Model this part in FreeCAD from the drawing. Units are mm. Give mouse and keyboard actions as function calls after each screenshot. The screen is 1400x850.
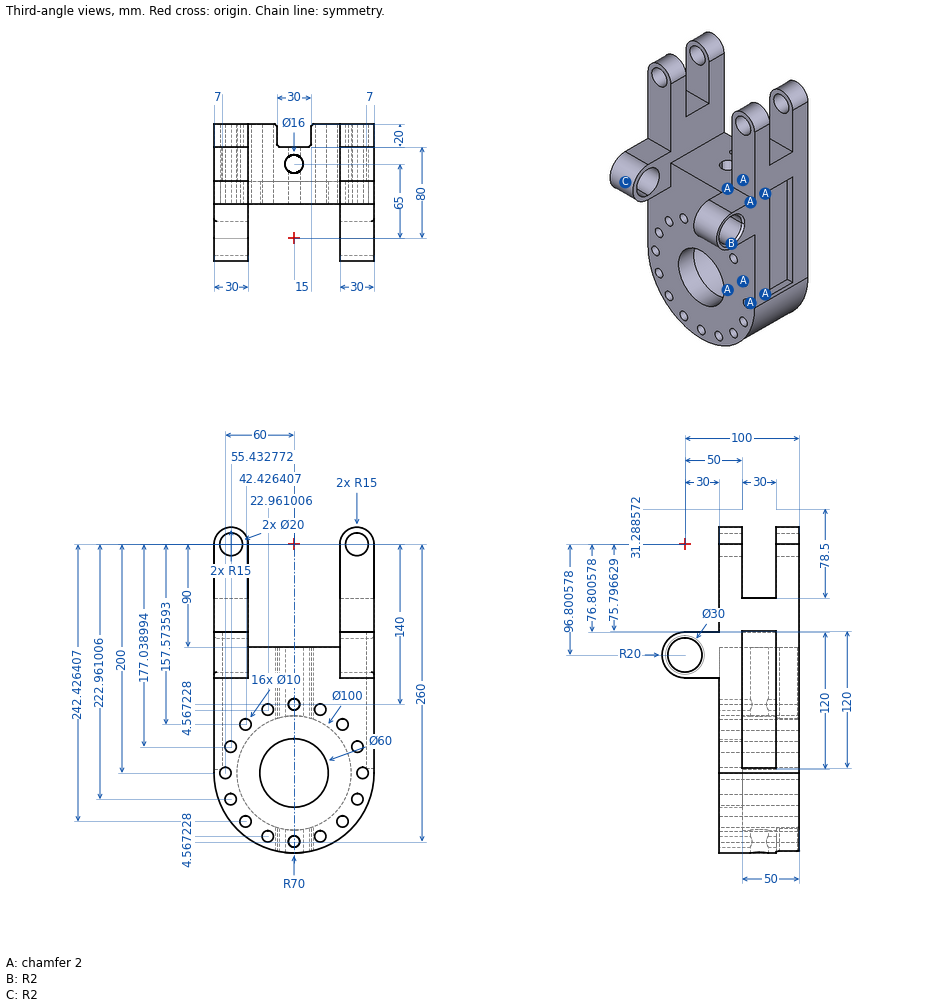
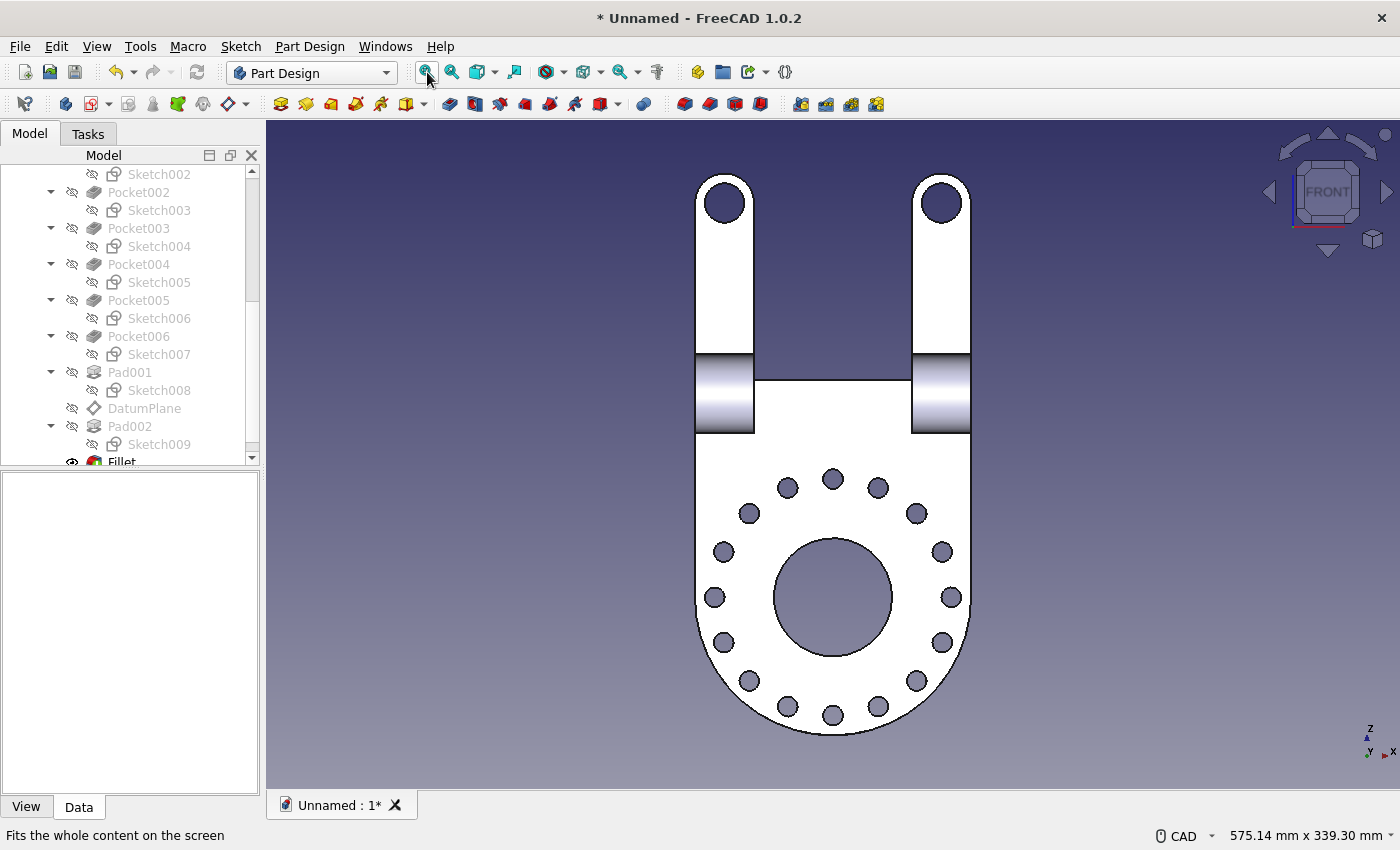
key(3)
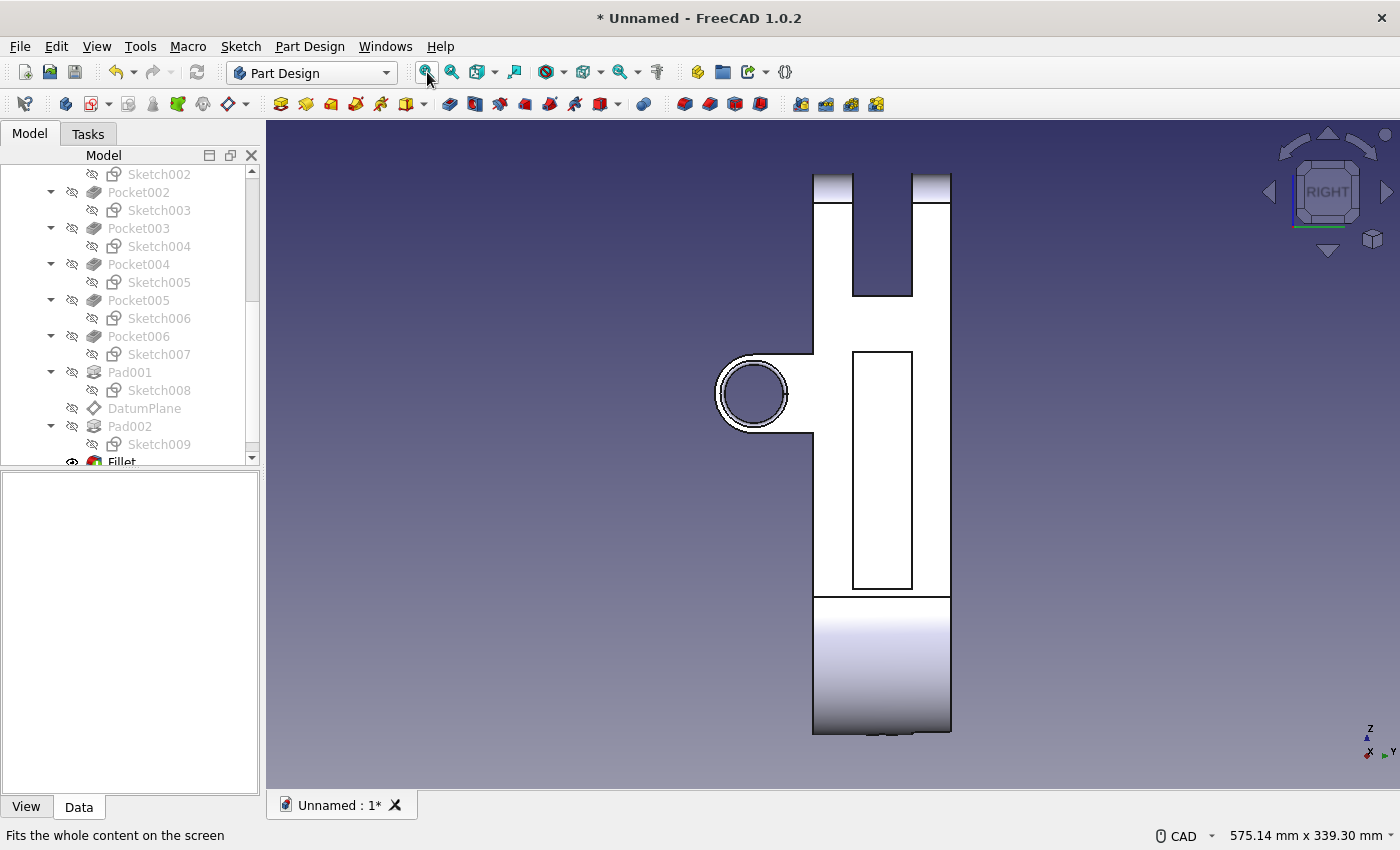
key(5)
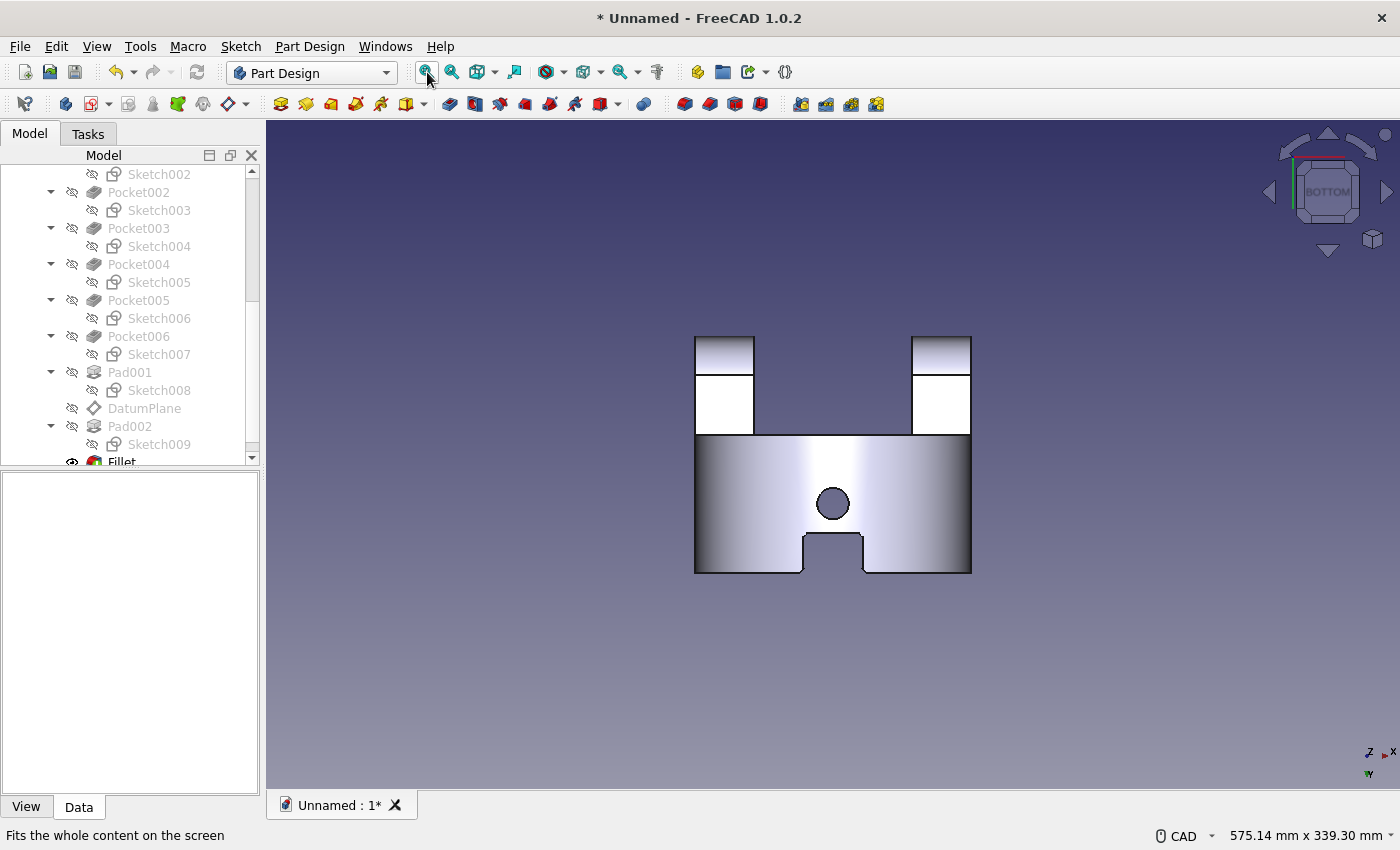
key(v)
key(f)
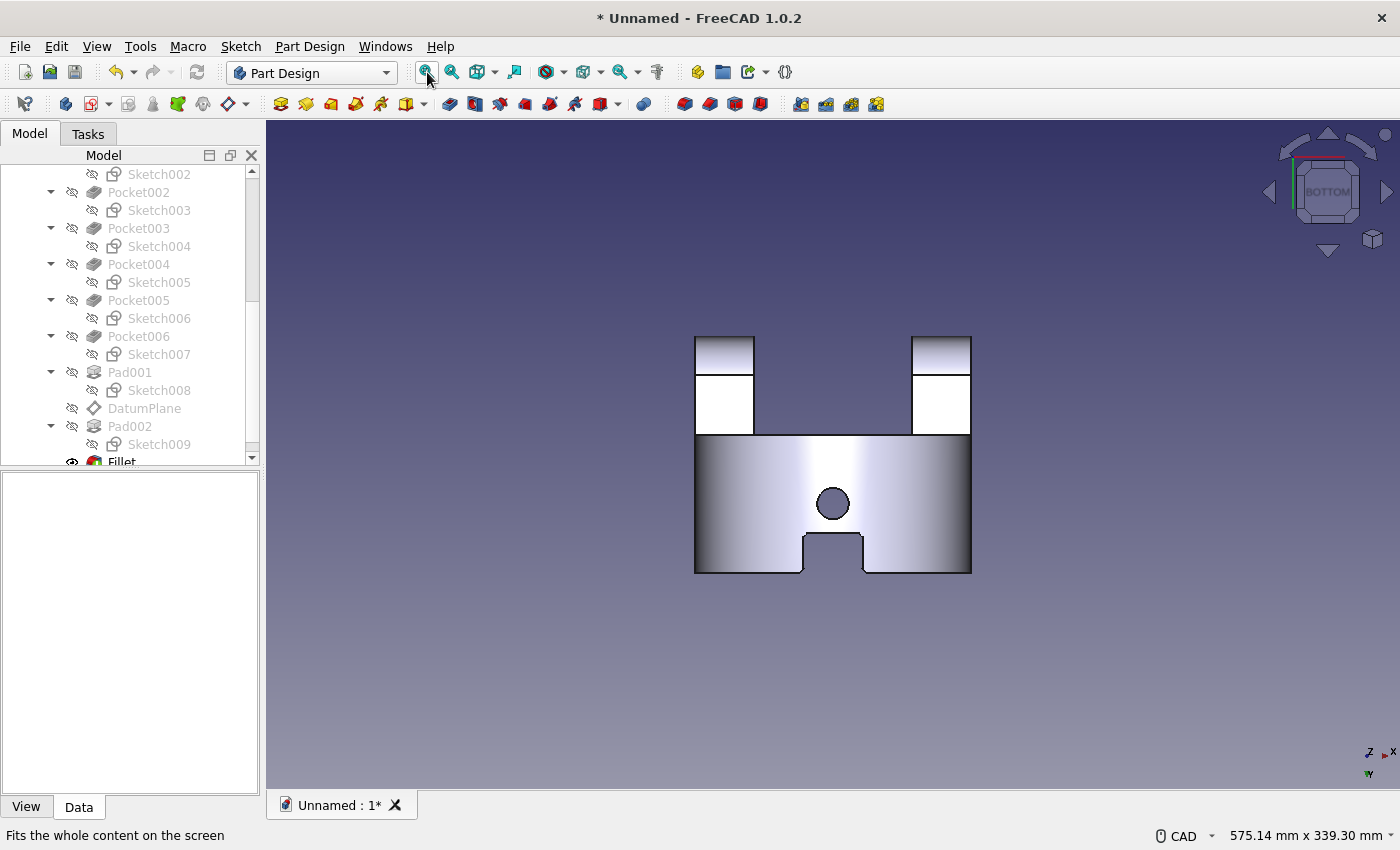
key(4)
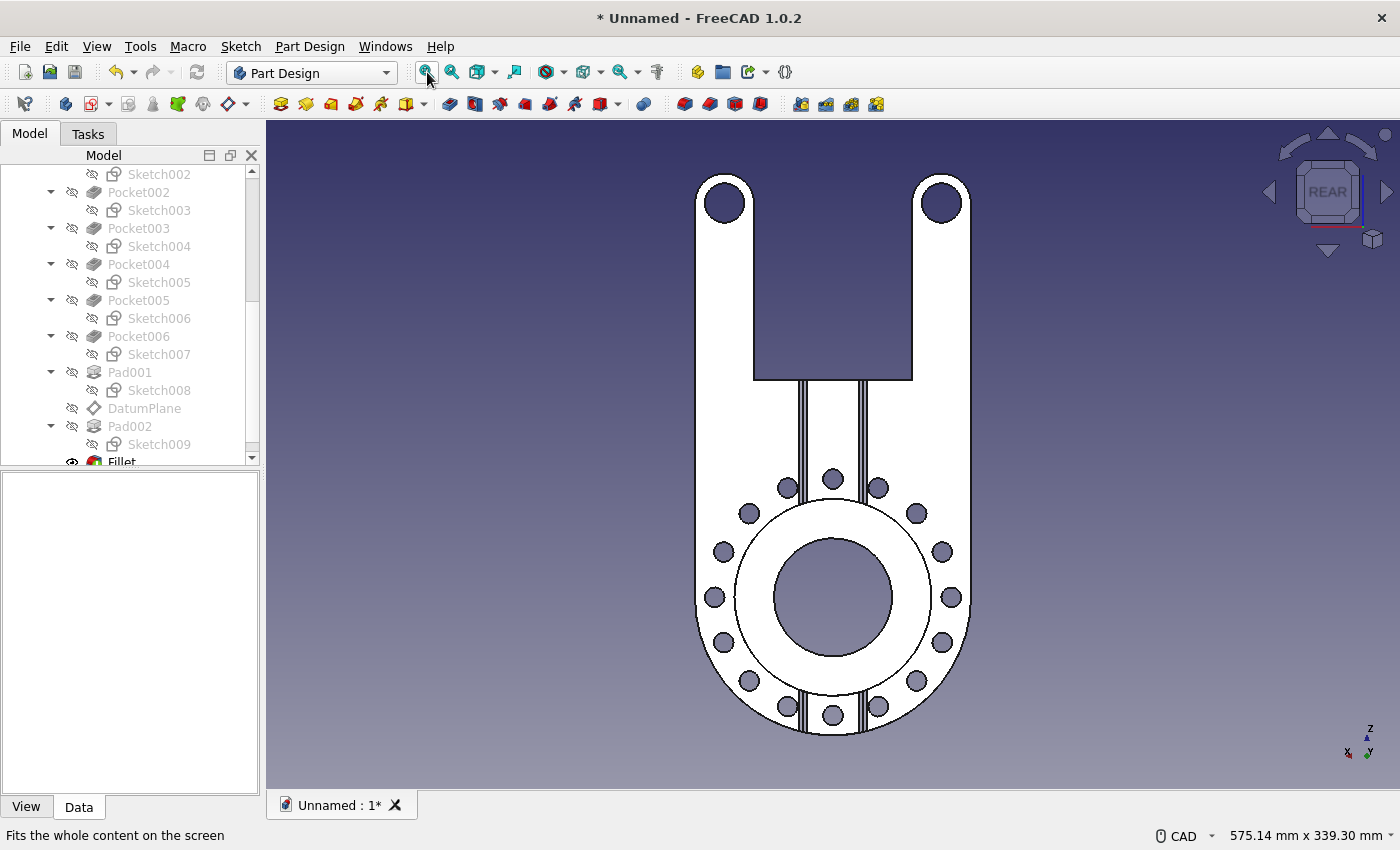
key(6)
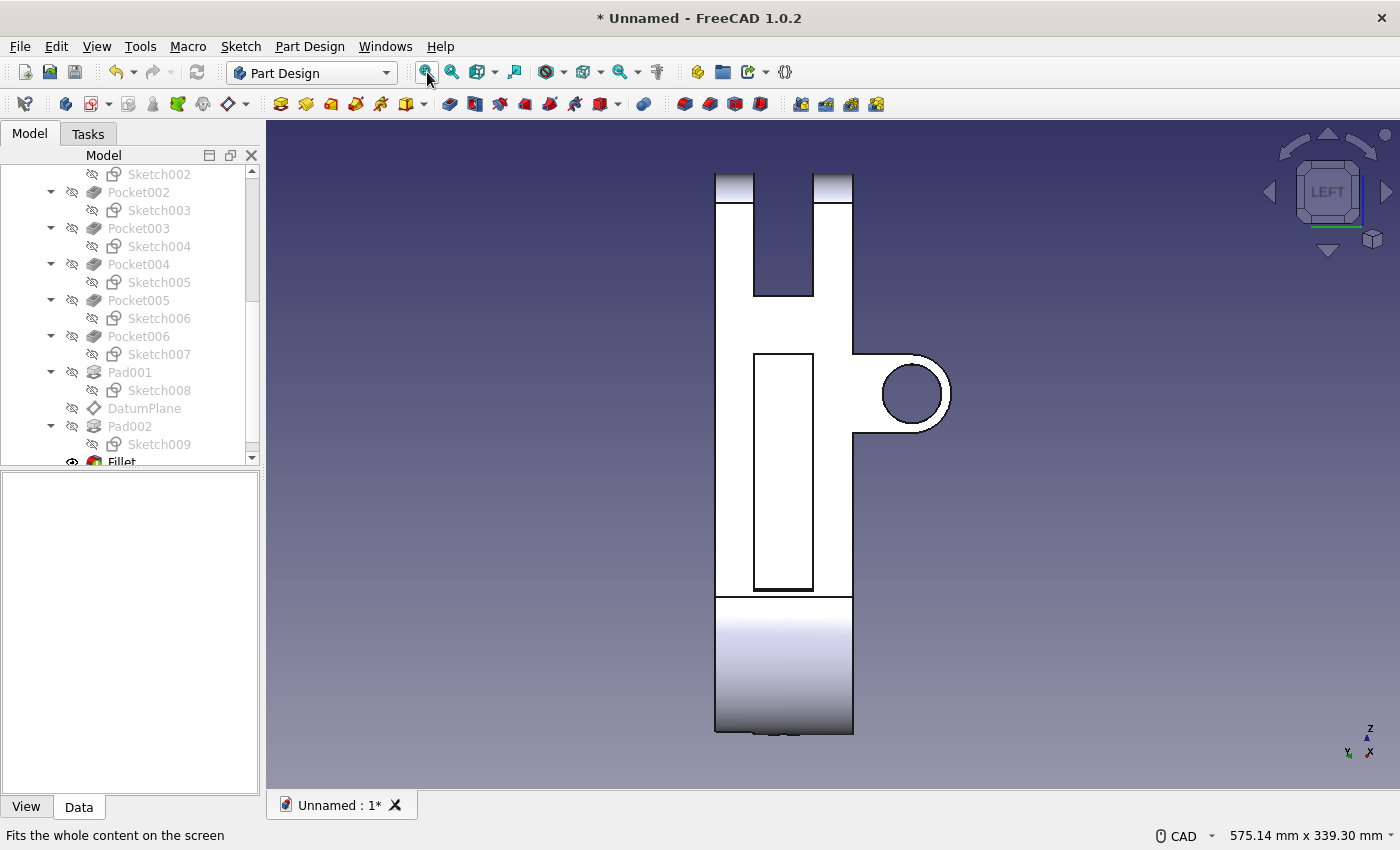
click(912, 363)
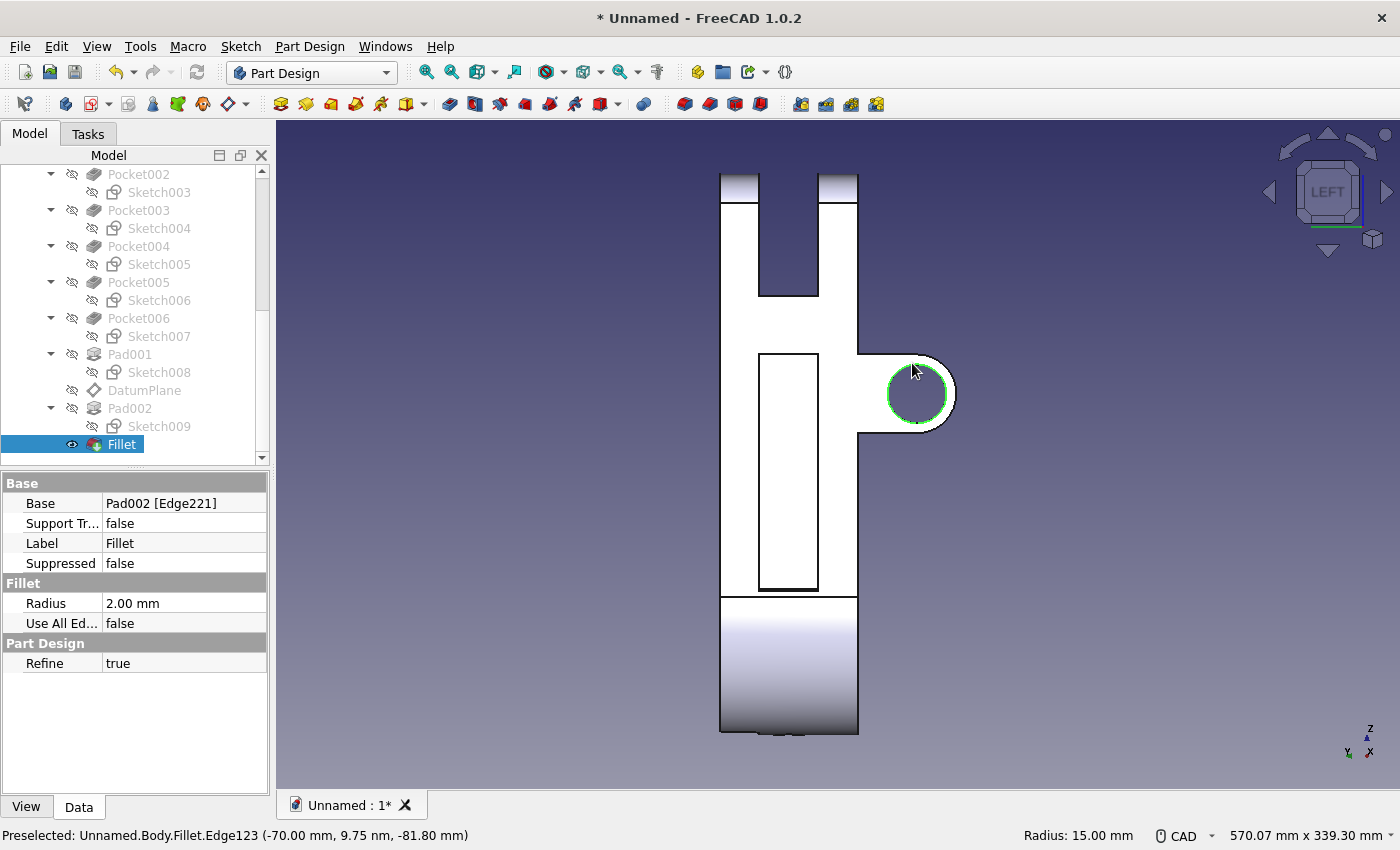
click(685, 104)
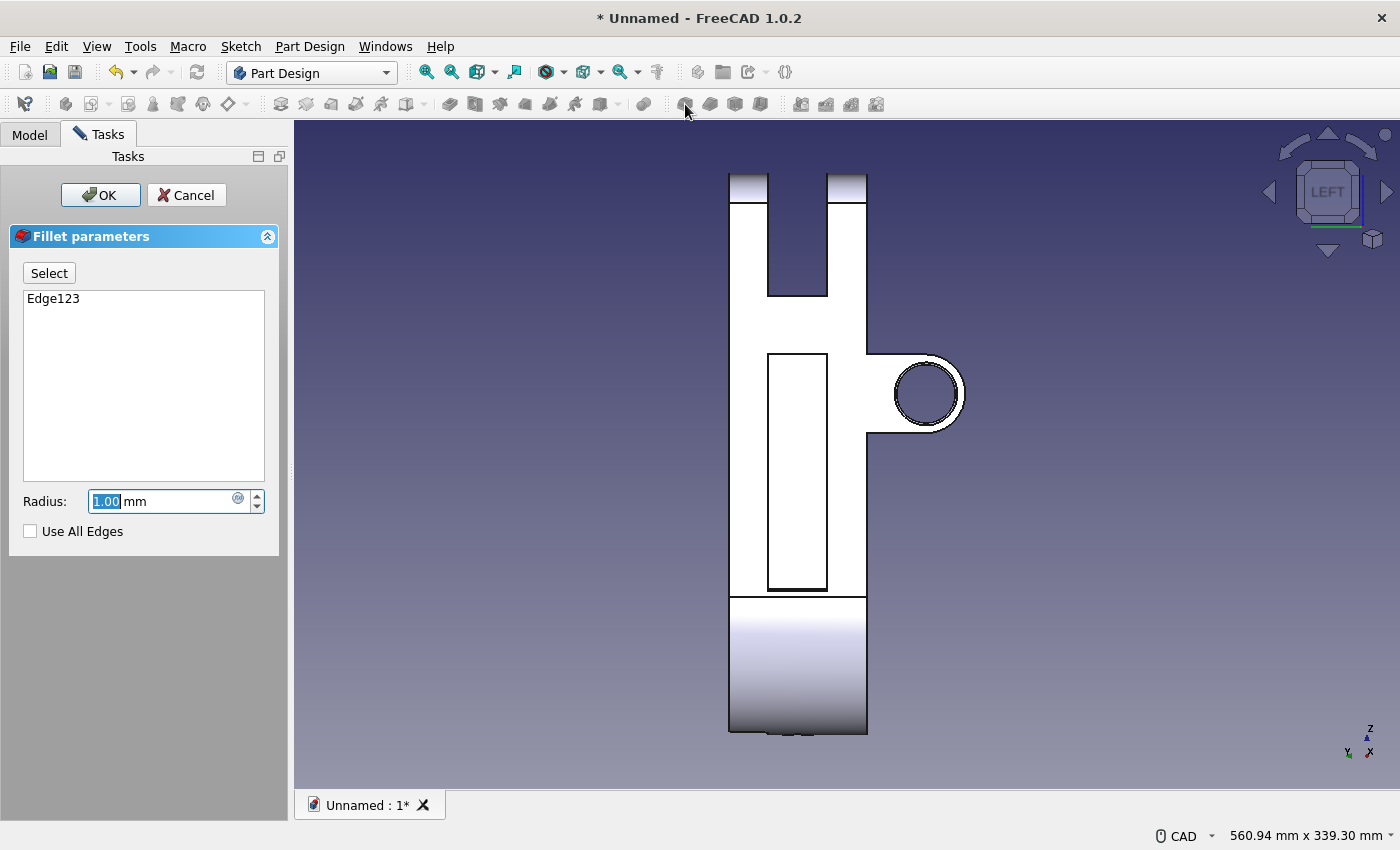
text(2)
key(Tab)